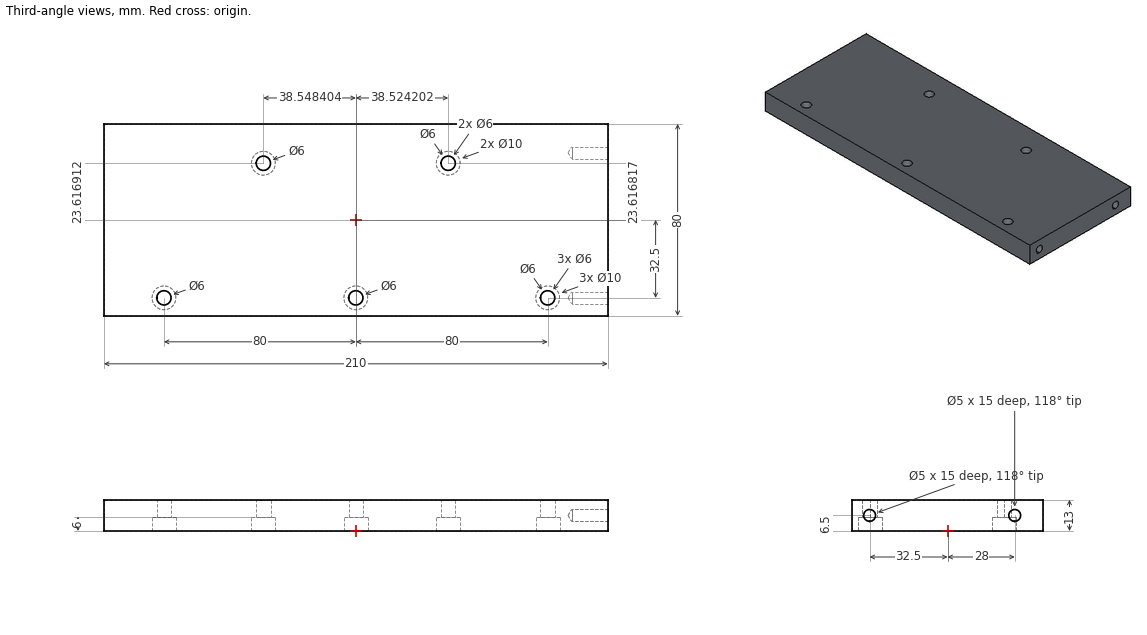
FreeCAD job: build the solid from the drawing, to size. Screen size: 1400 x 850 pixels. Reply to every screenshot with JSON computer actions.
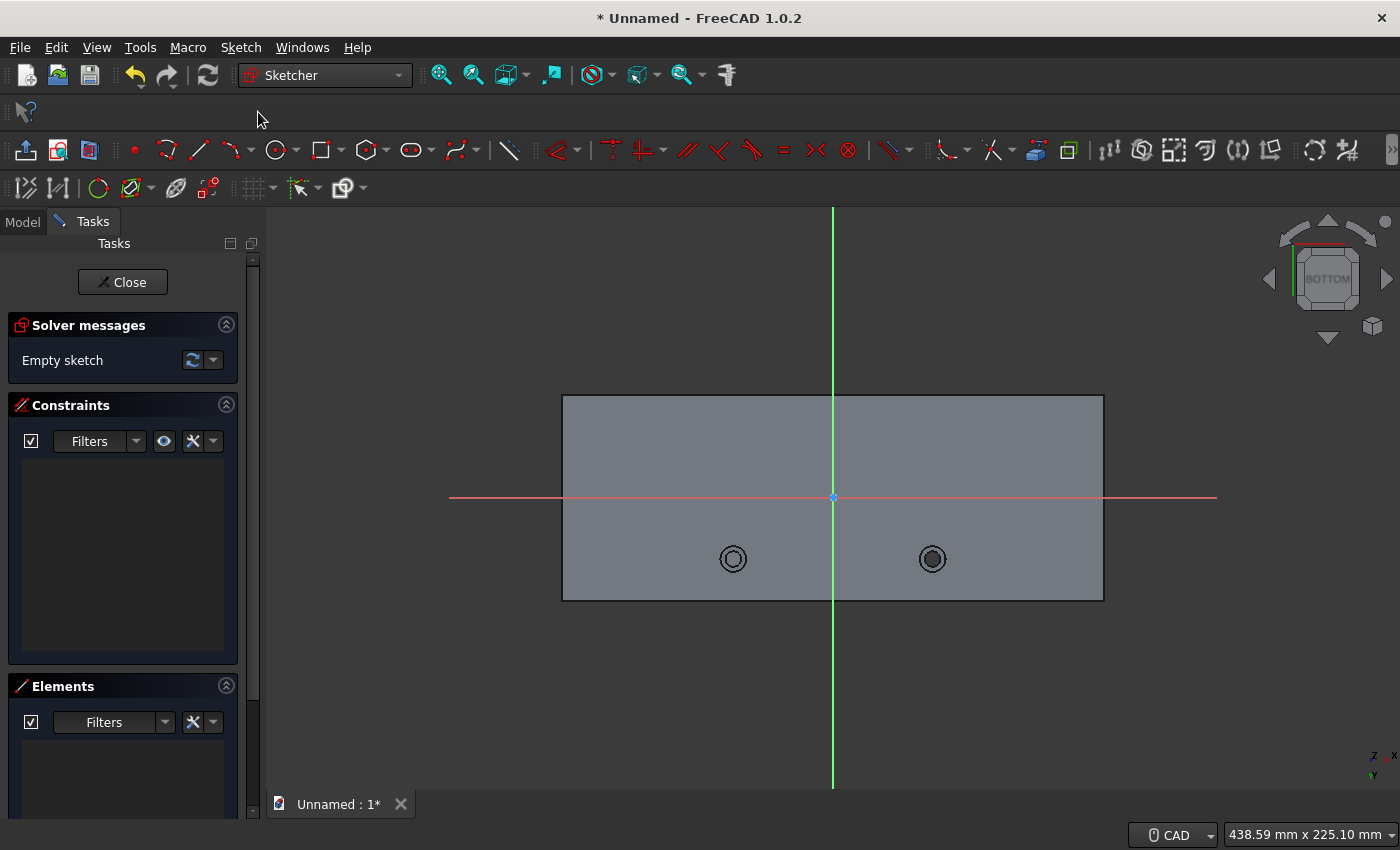
{"action": "scroll", "coordinate": [732, 562], "scroll_direction": "up", "scroll_amount": 15}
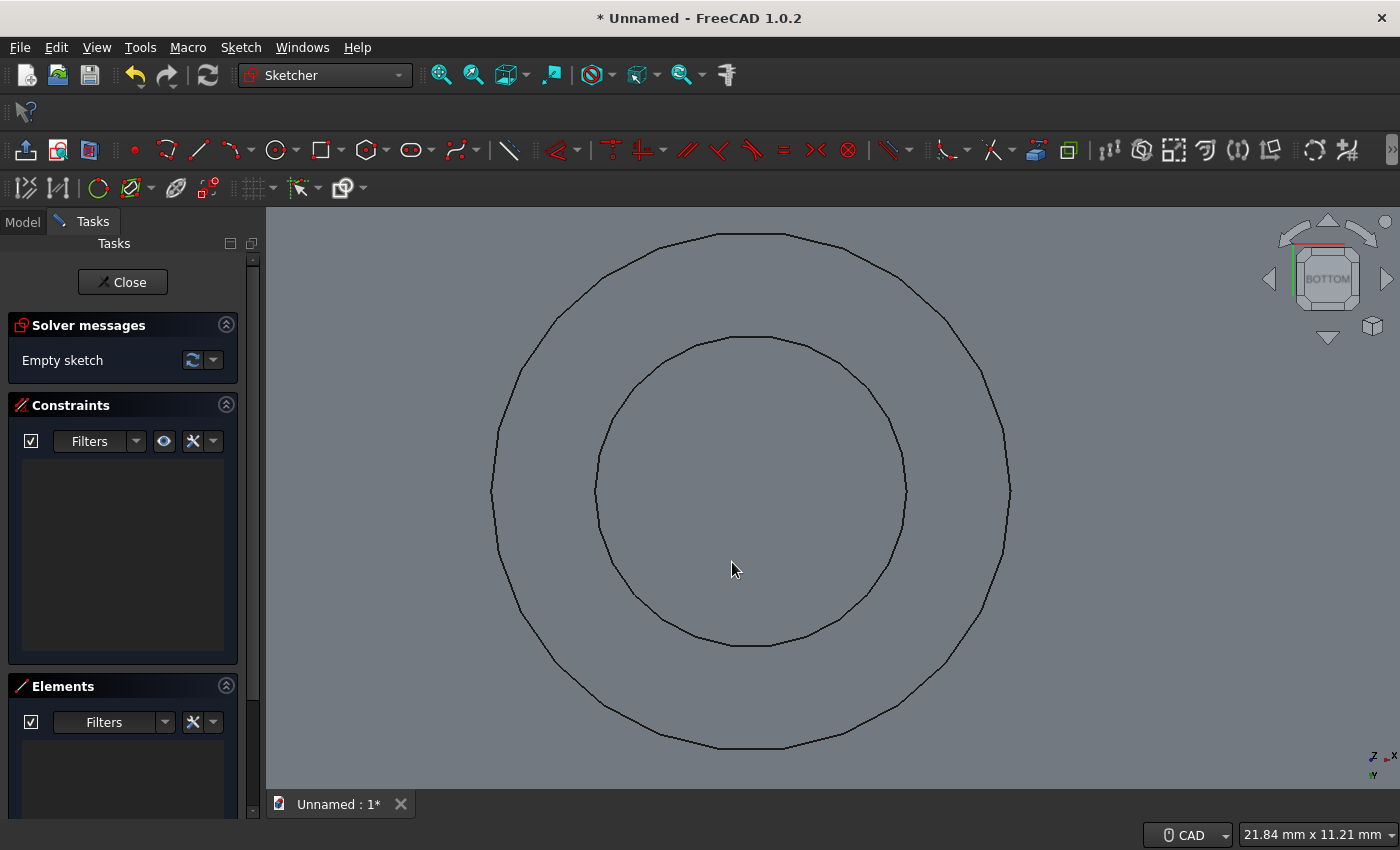
{"action": "key", "text": "g c"}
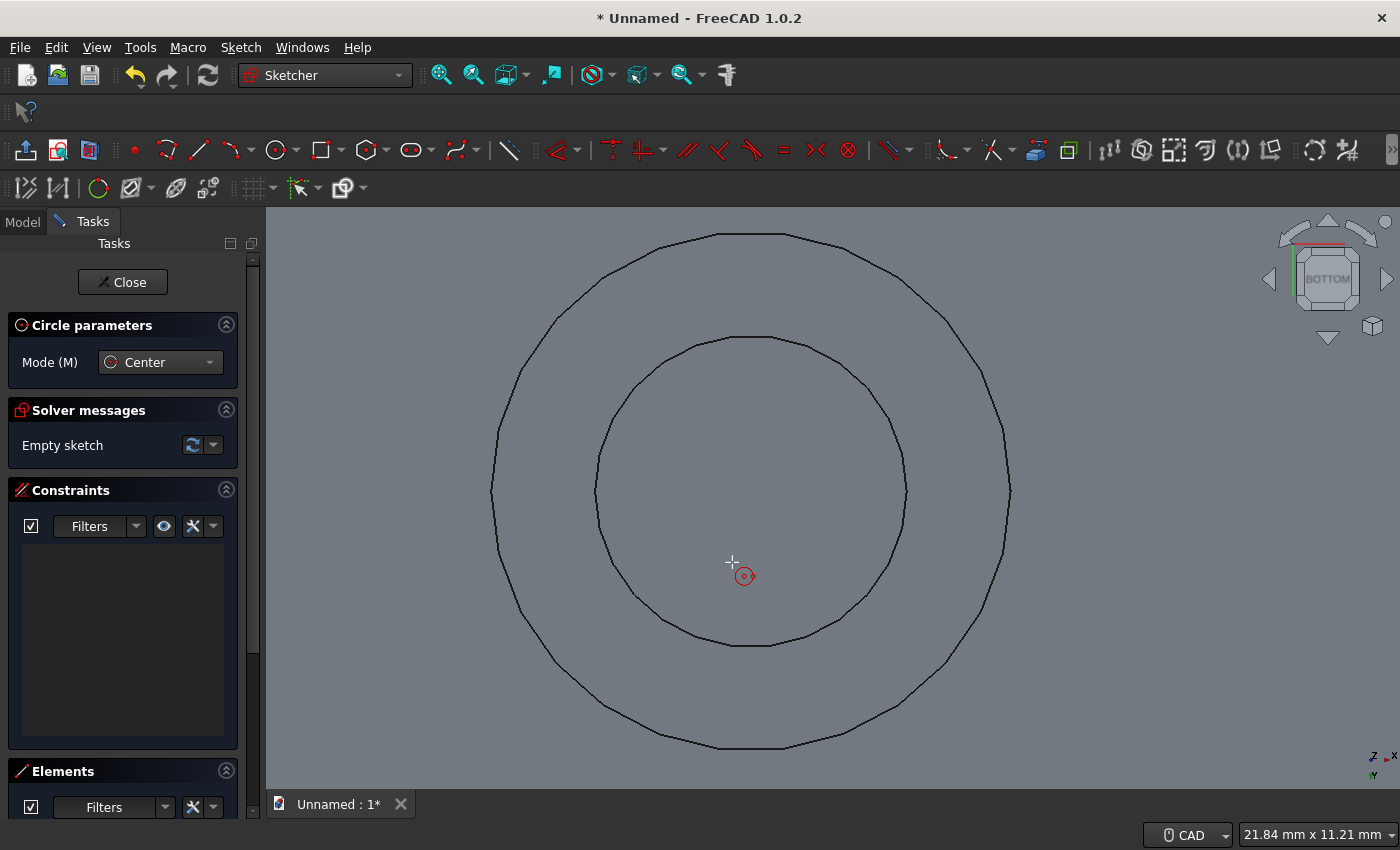
{"action": "left_click", "coordinate": [751, 491]}
{"action": "left_click", "coordinate": [861, 381]}
{"action": "key", "text": "Escape"}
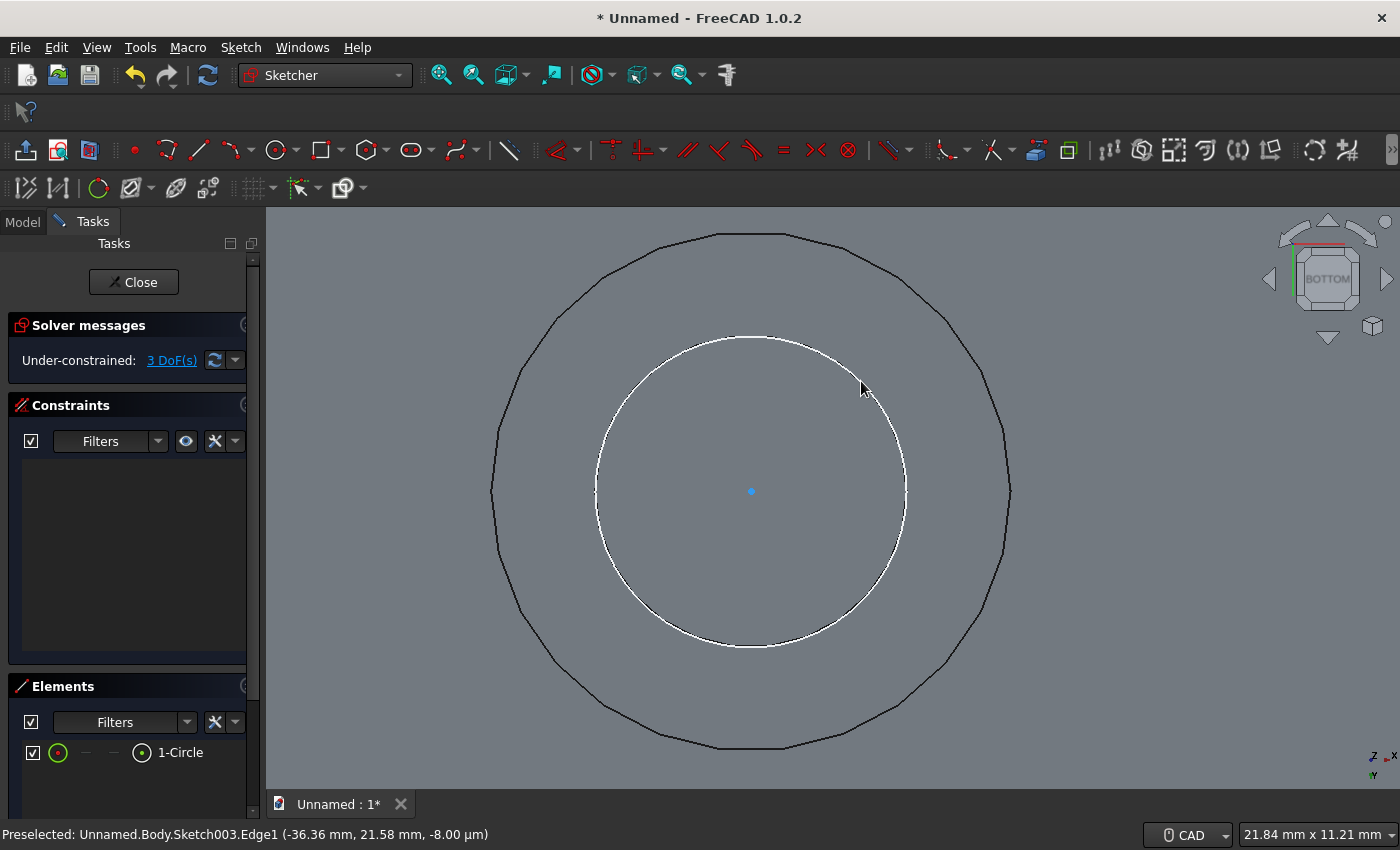
{"action": "key", "text": "d"}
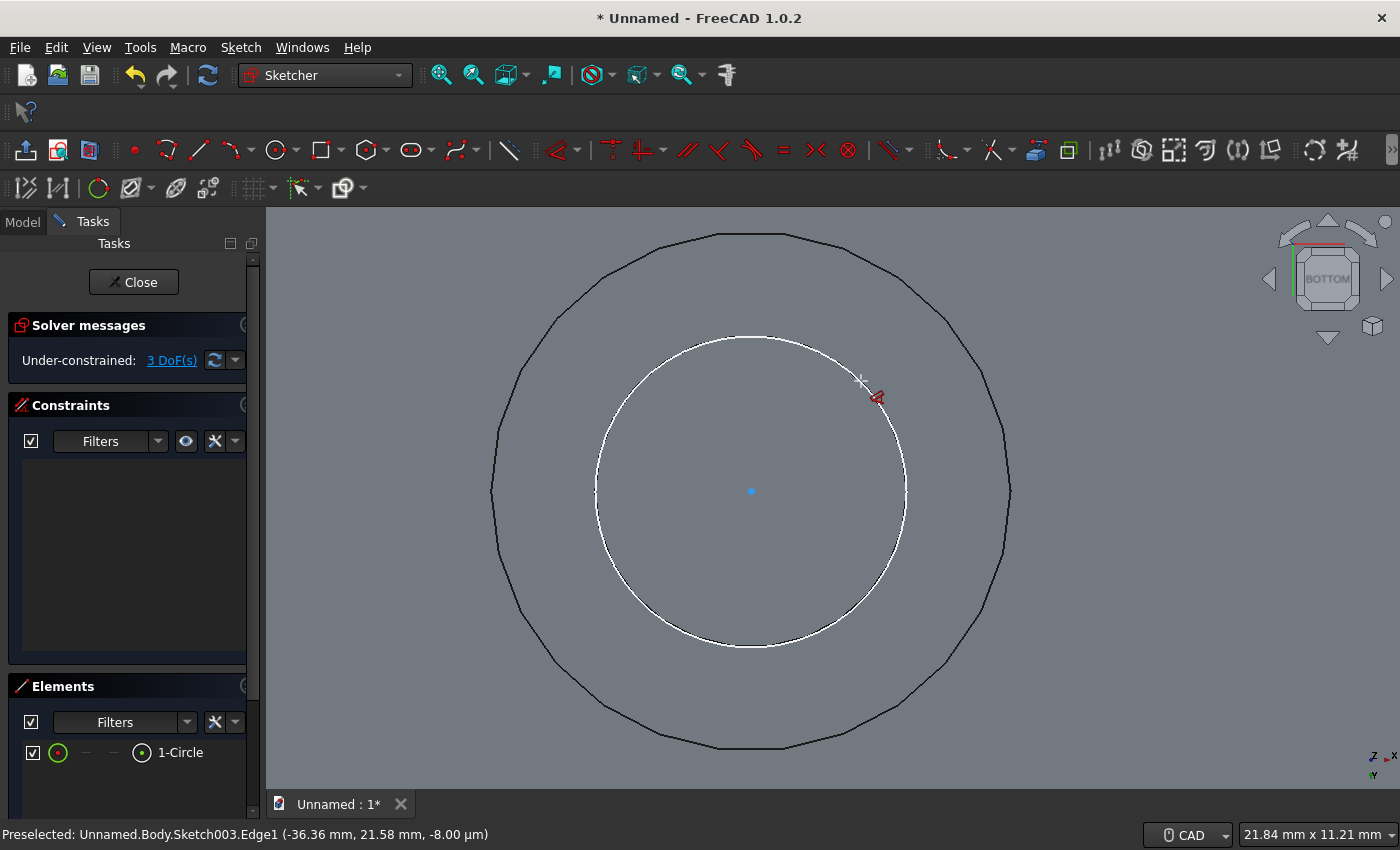
{"action": "left_click", "coordinate": [861, 382]}
{"action": "left_click", "coordinate": [884, 359]}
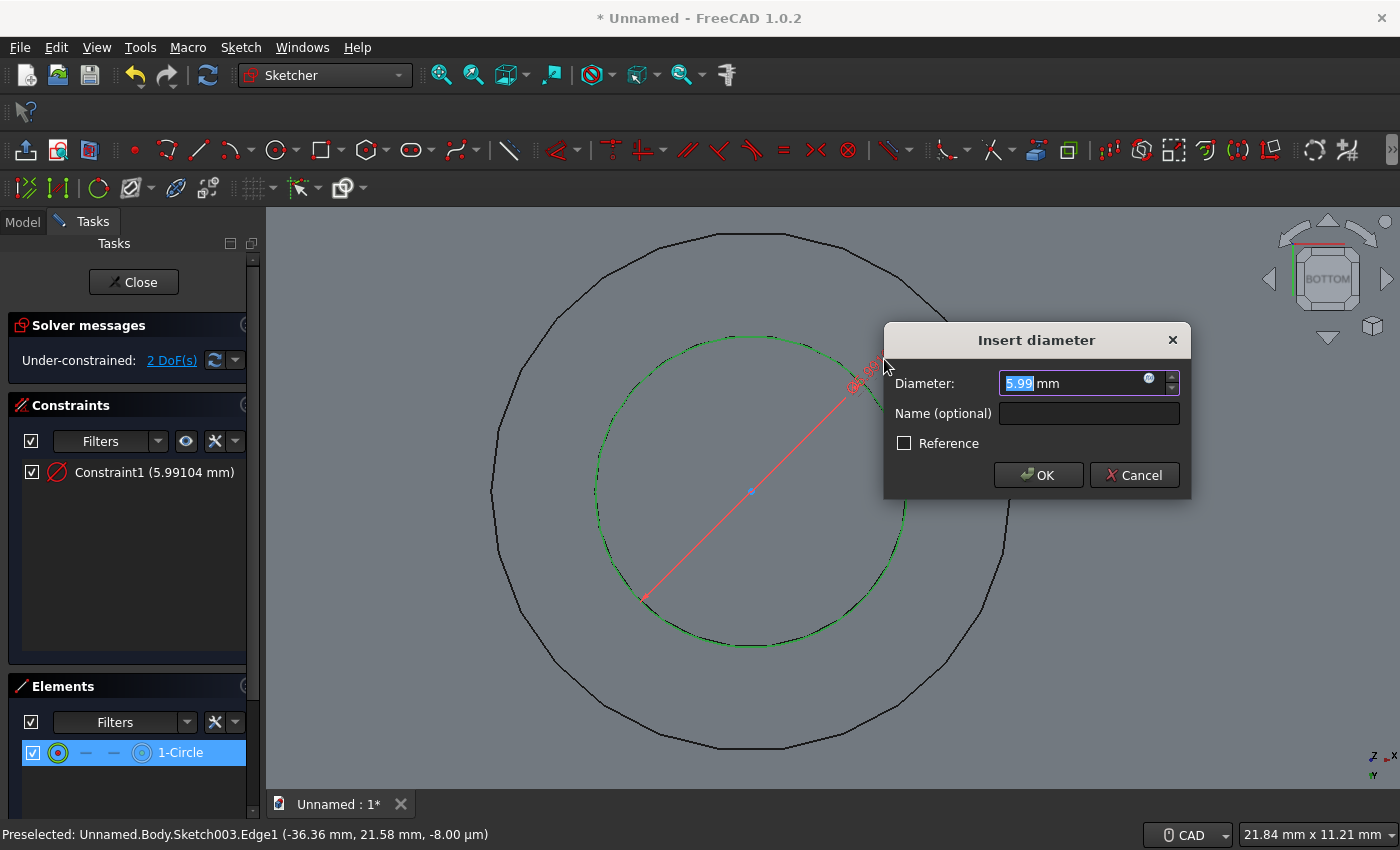
{"action": "type", "text": "6"}
{"action": "key", "text": "Return"}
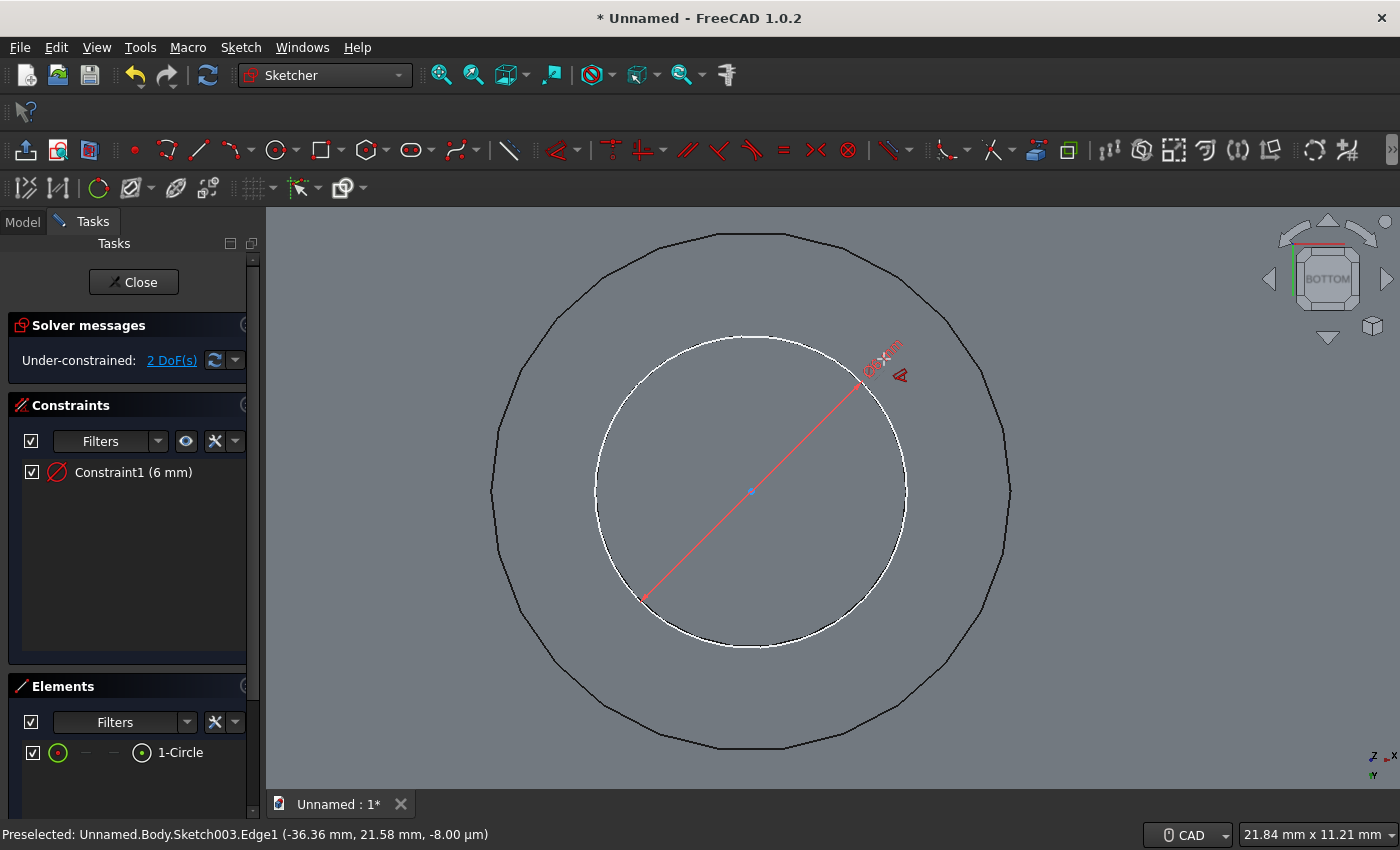
{"action": "left_click", "coordinate": [751, 492]}
{"action": "left_click", "coordinate": [993, 526]}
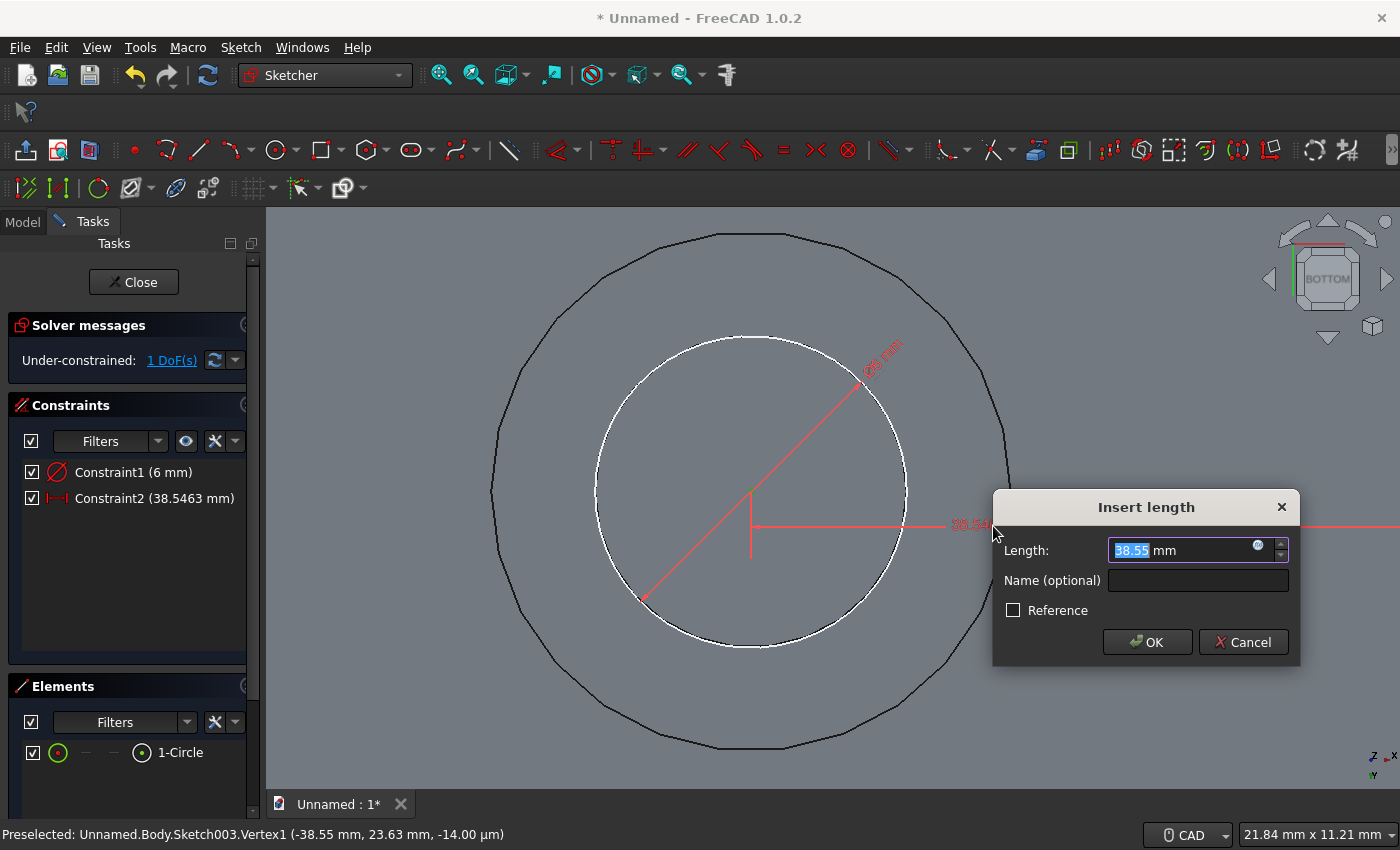
{"action": "type", "text": "38.548404"}
{"action": "key", "text": "Return"}